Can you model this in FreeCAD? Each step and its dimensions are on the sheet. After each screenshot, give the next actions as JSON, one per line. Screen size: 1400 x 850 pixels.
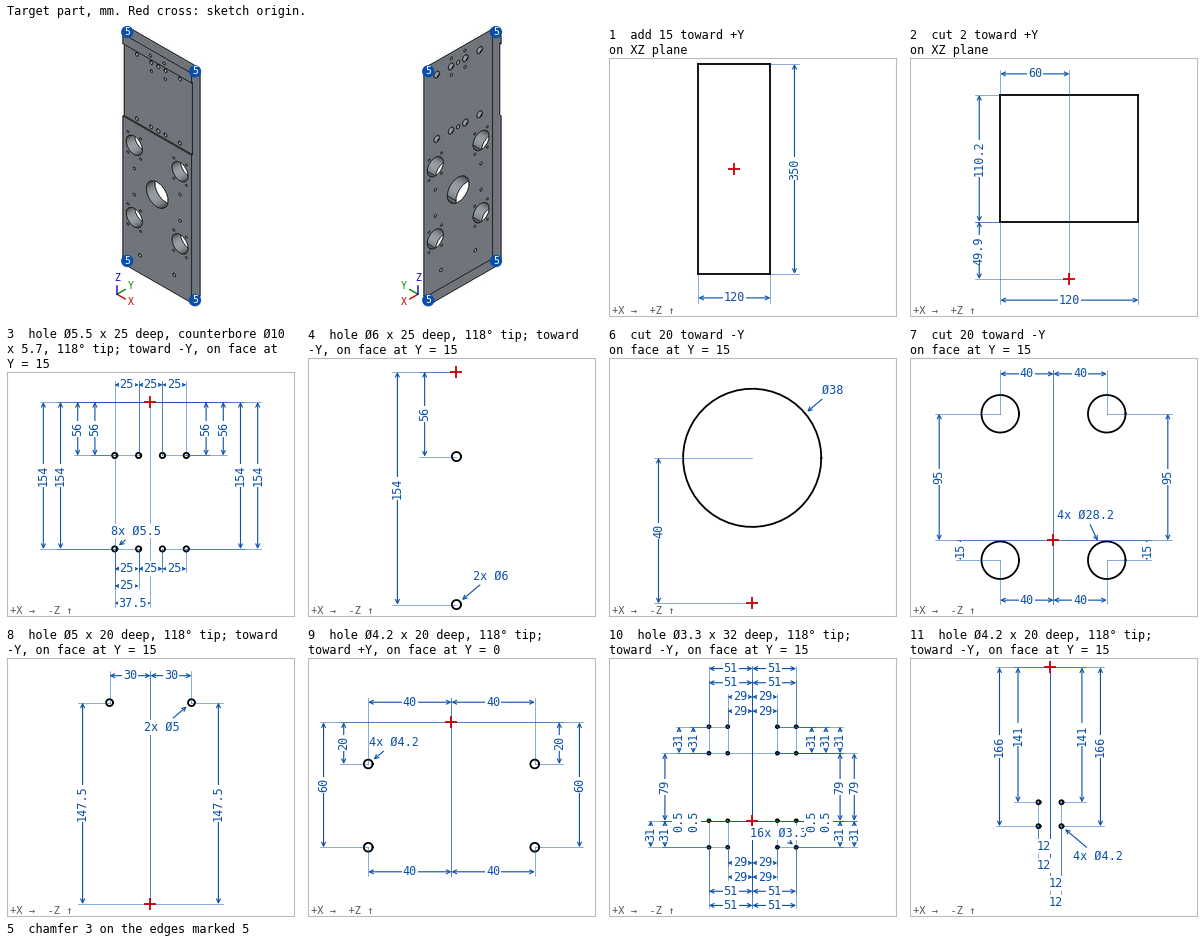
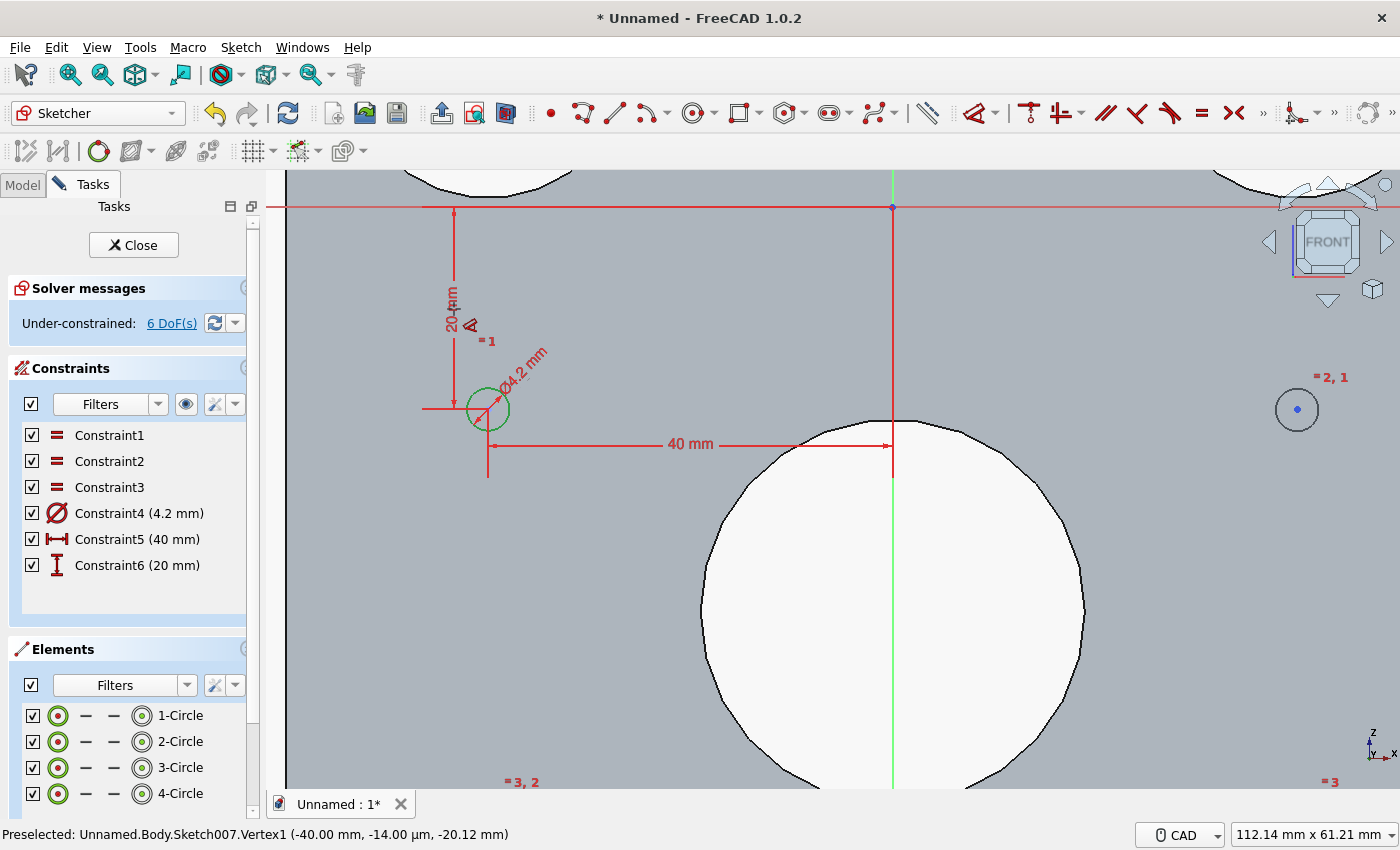
{"action": "scroll", "coordinate": [504, 395], "scroll_direction": "down", "scroll_amount": 2}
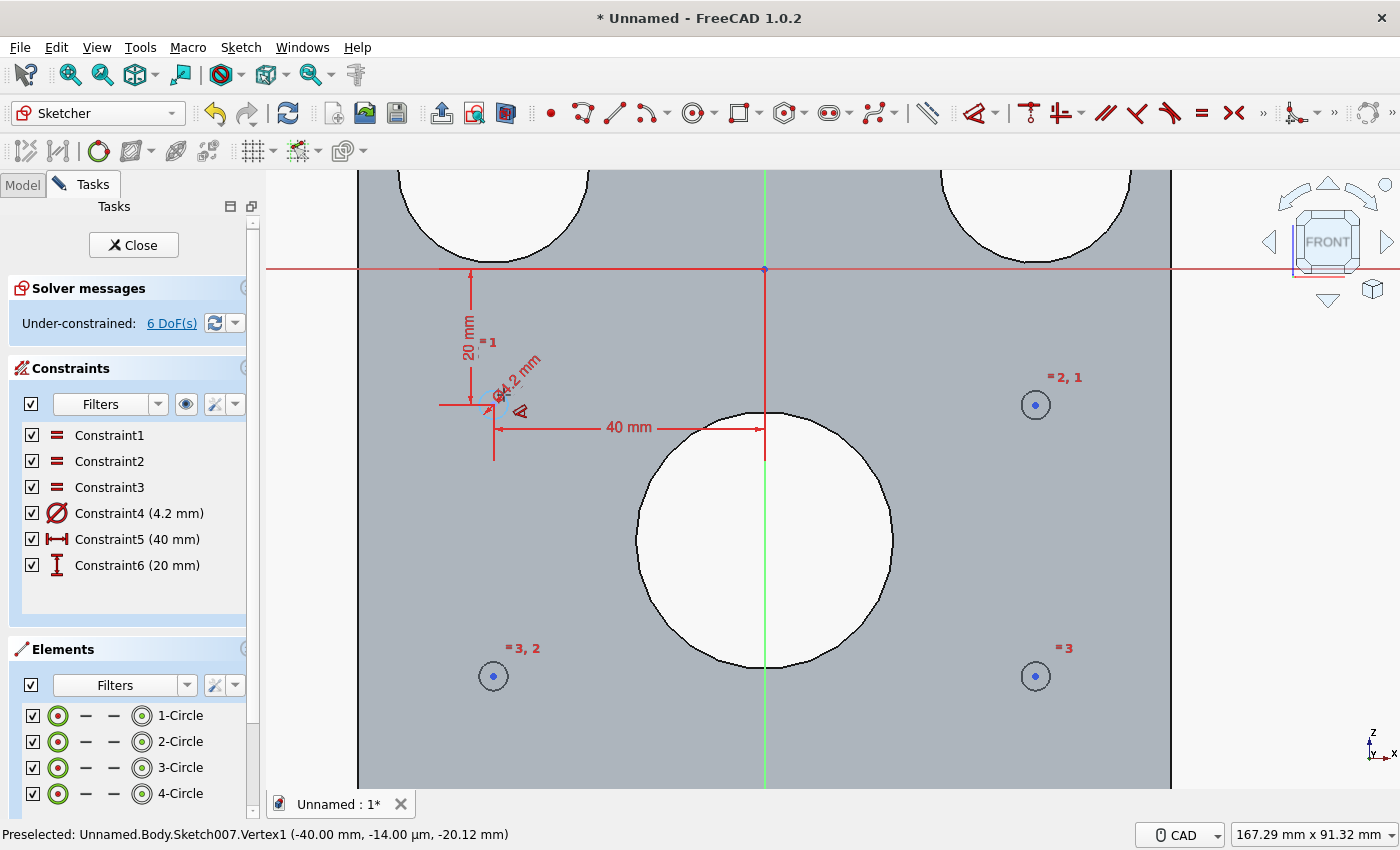
{"action": "left_click", "coordinate": [1036, 405]}
{"action": "left_click", "coordinate": [900, 235]}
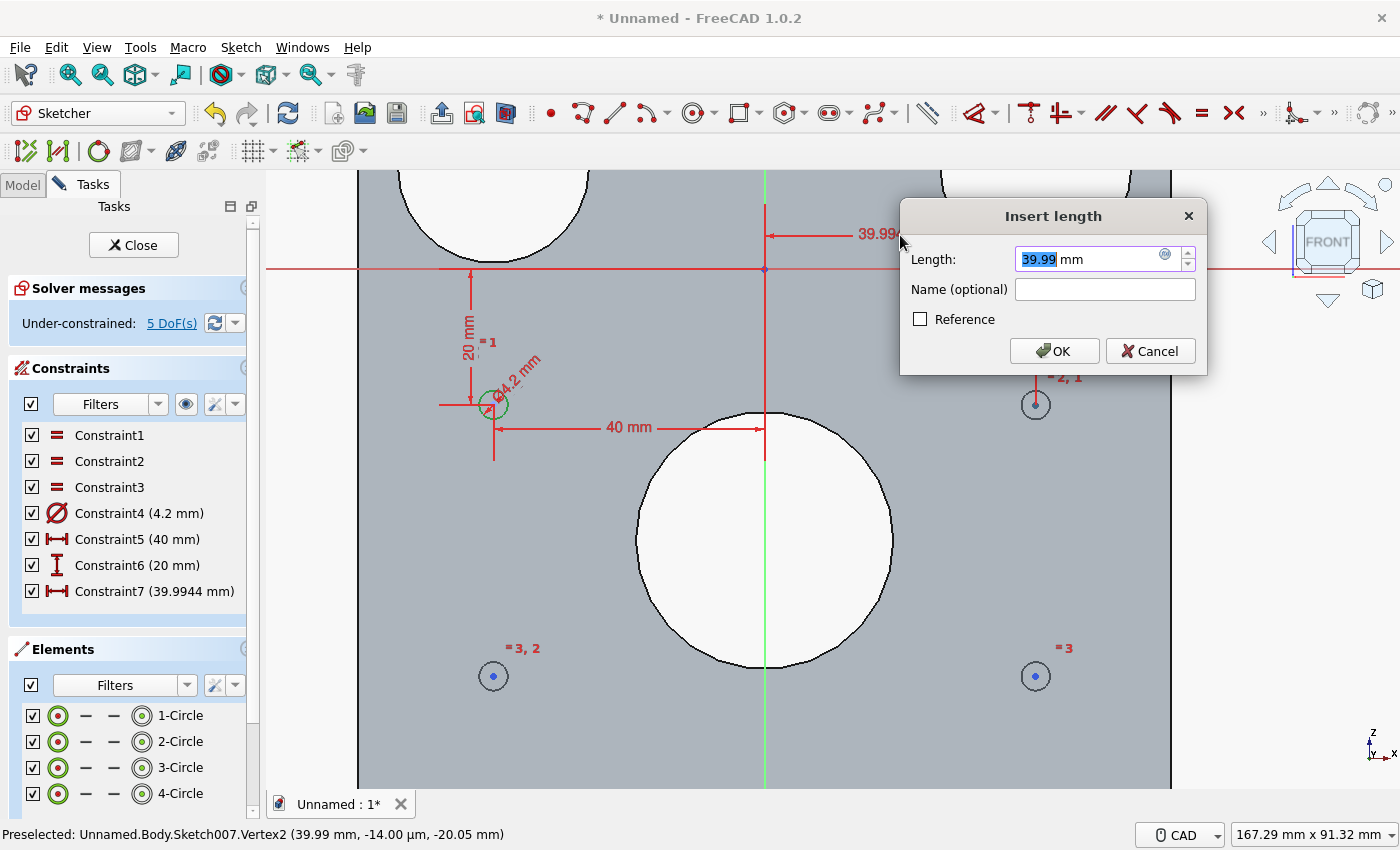
{"action": "type", "text": "40"}
{"action": "key", "text": "Return"}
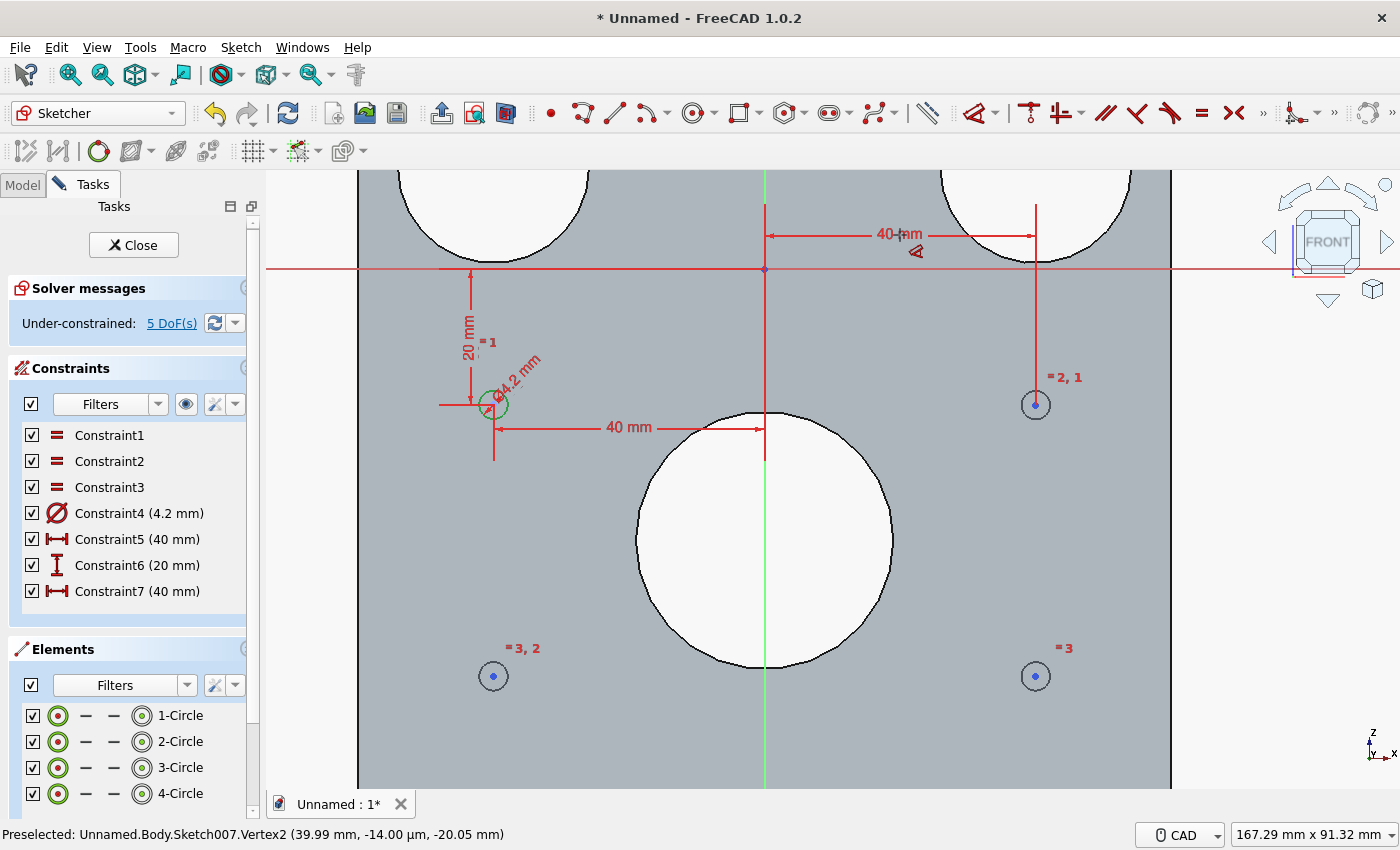
{"action": "left_click", "coordinate": [1036, 405]}
{"action": "left_click", "coordinate": [1070, 337]}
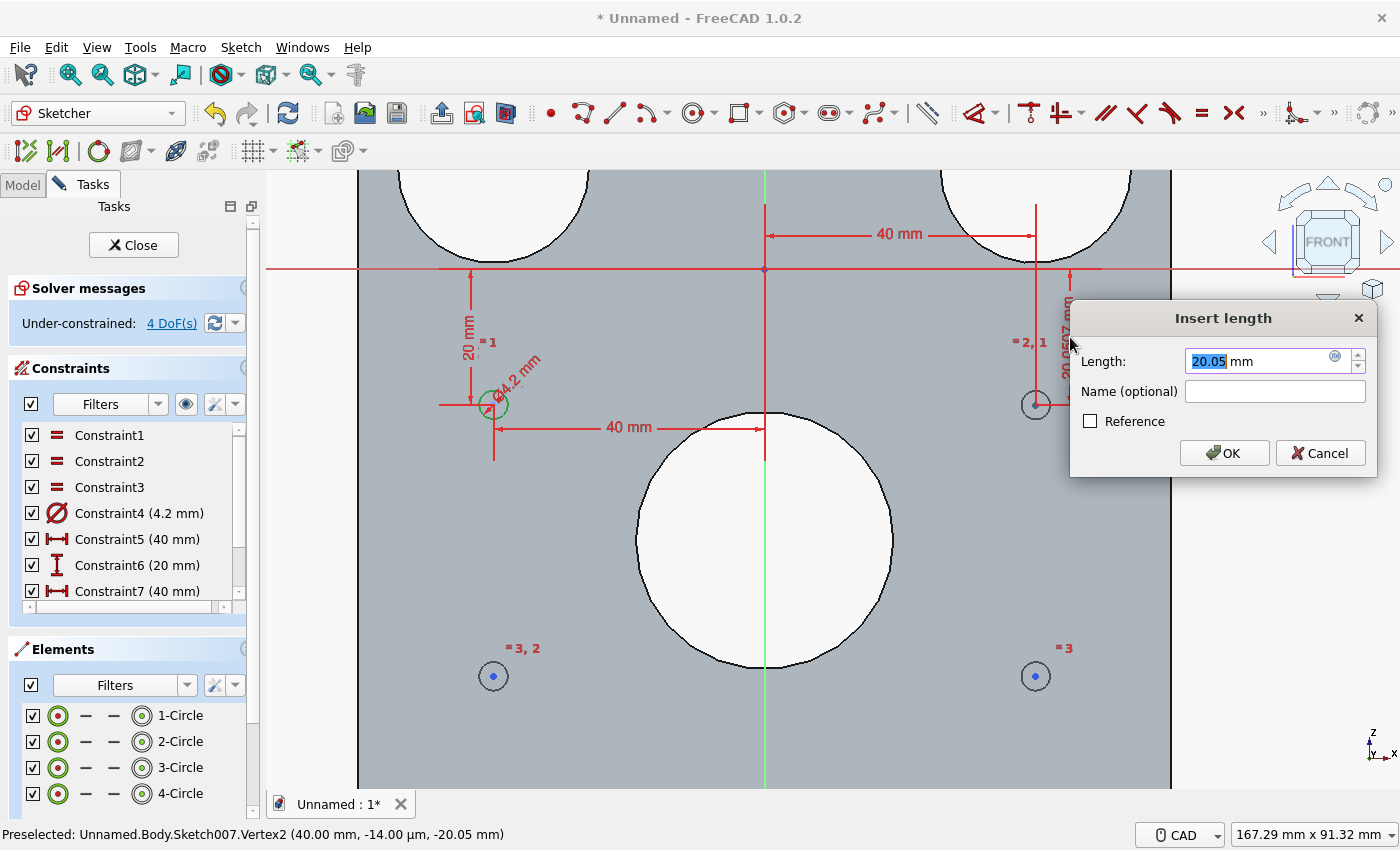
{"action": "type", "text": "20"}
{"action": "key", "text": "Return"}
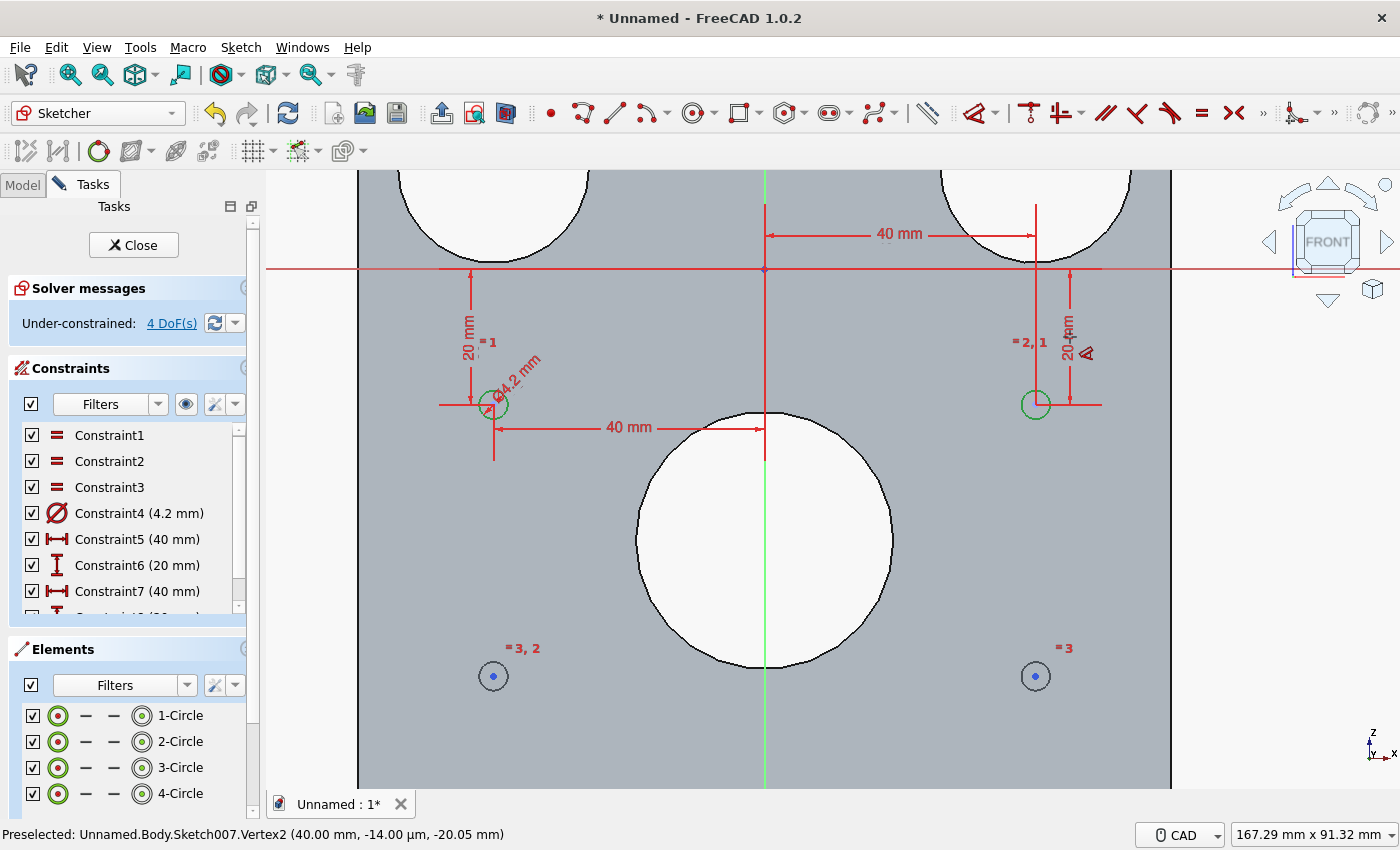
{"action": "left_click", "coordinate": [494, 676]}
{"action": "left_click", "coordinate": [629, 235]}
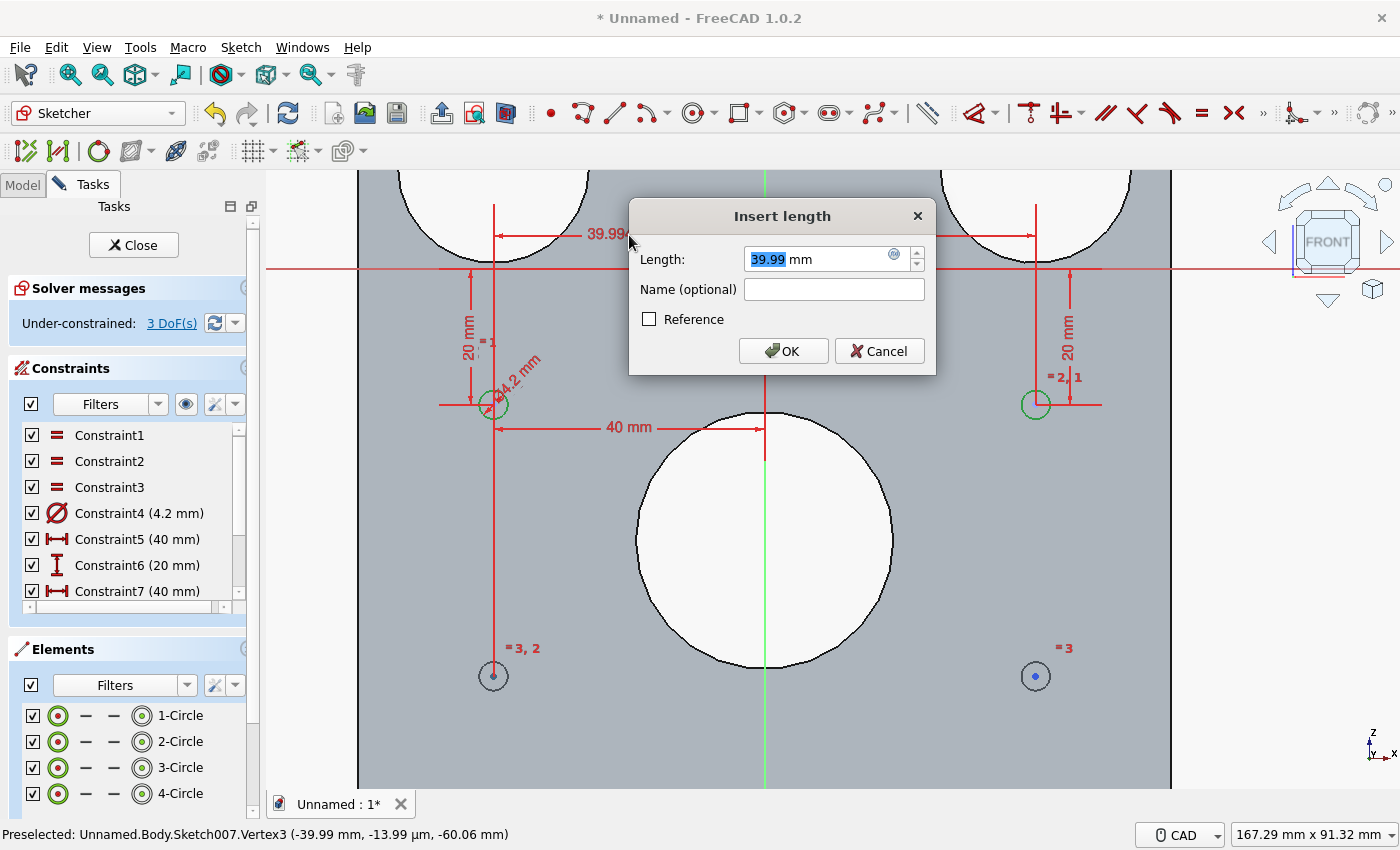
{"action": "type", "text": "40"}
{"action": "key", "text": "Return"}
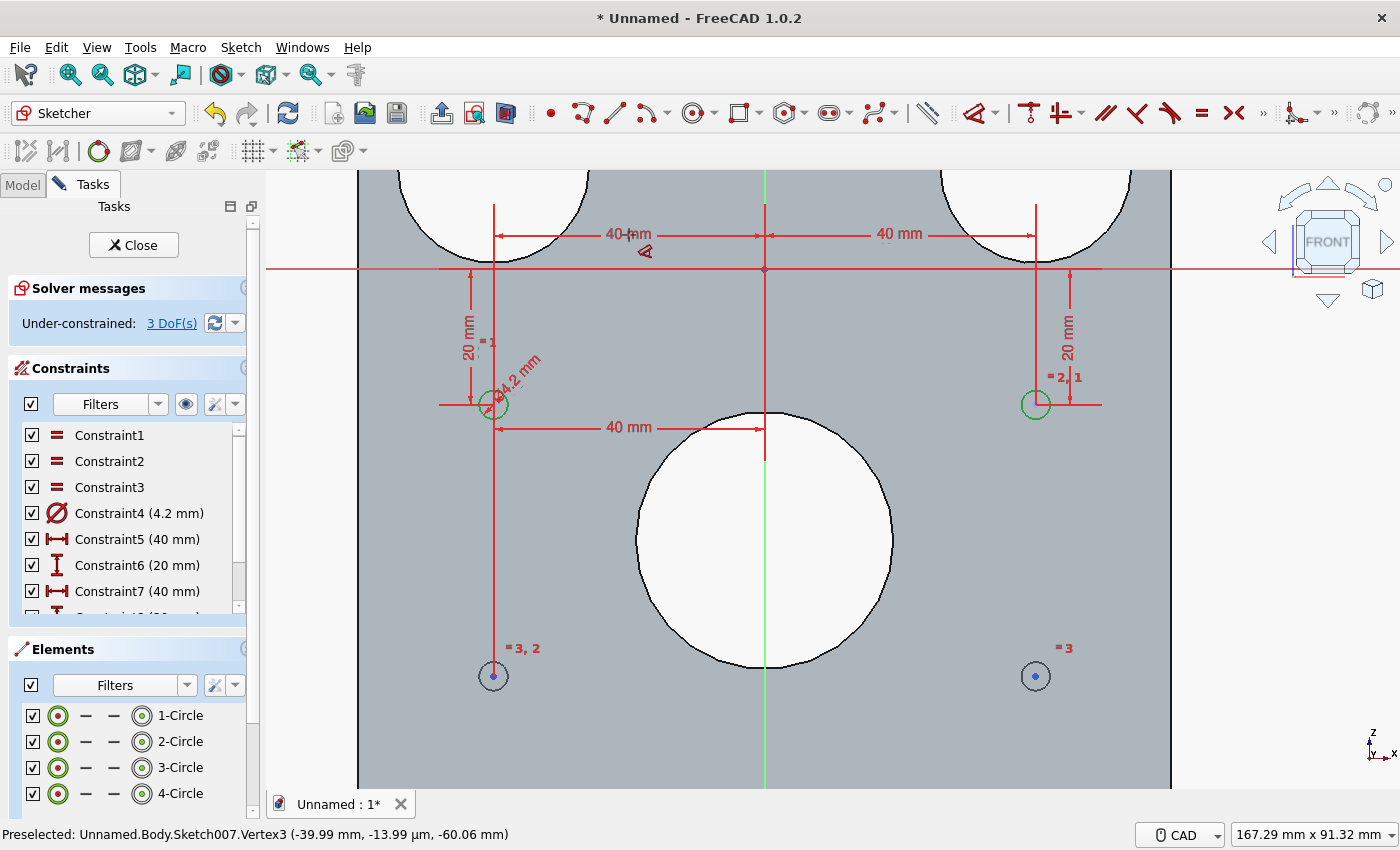
{"action": "left_click", "coordinate": [494, 676]}
{"action": "left_click", "coordinate": [460, 473]}